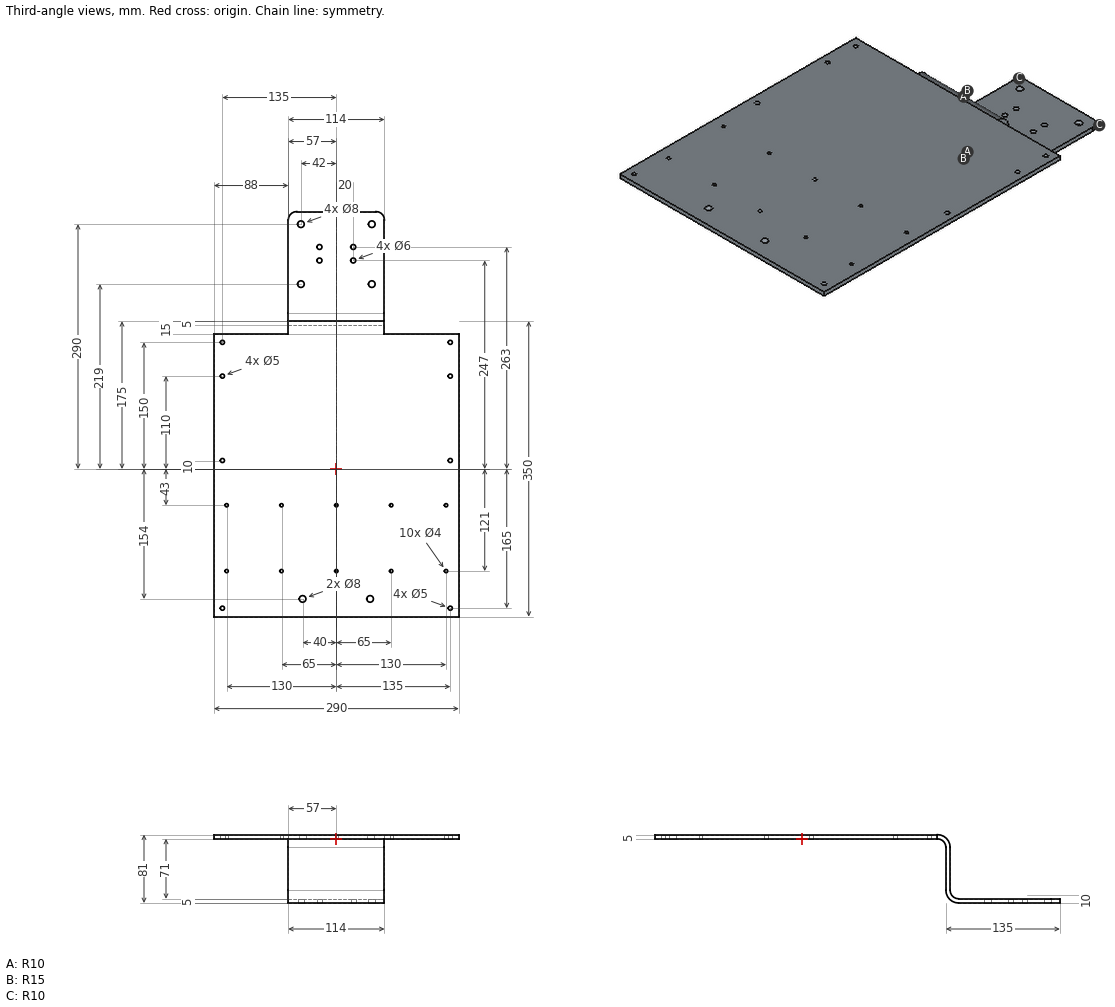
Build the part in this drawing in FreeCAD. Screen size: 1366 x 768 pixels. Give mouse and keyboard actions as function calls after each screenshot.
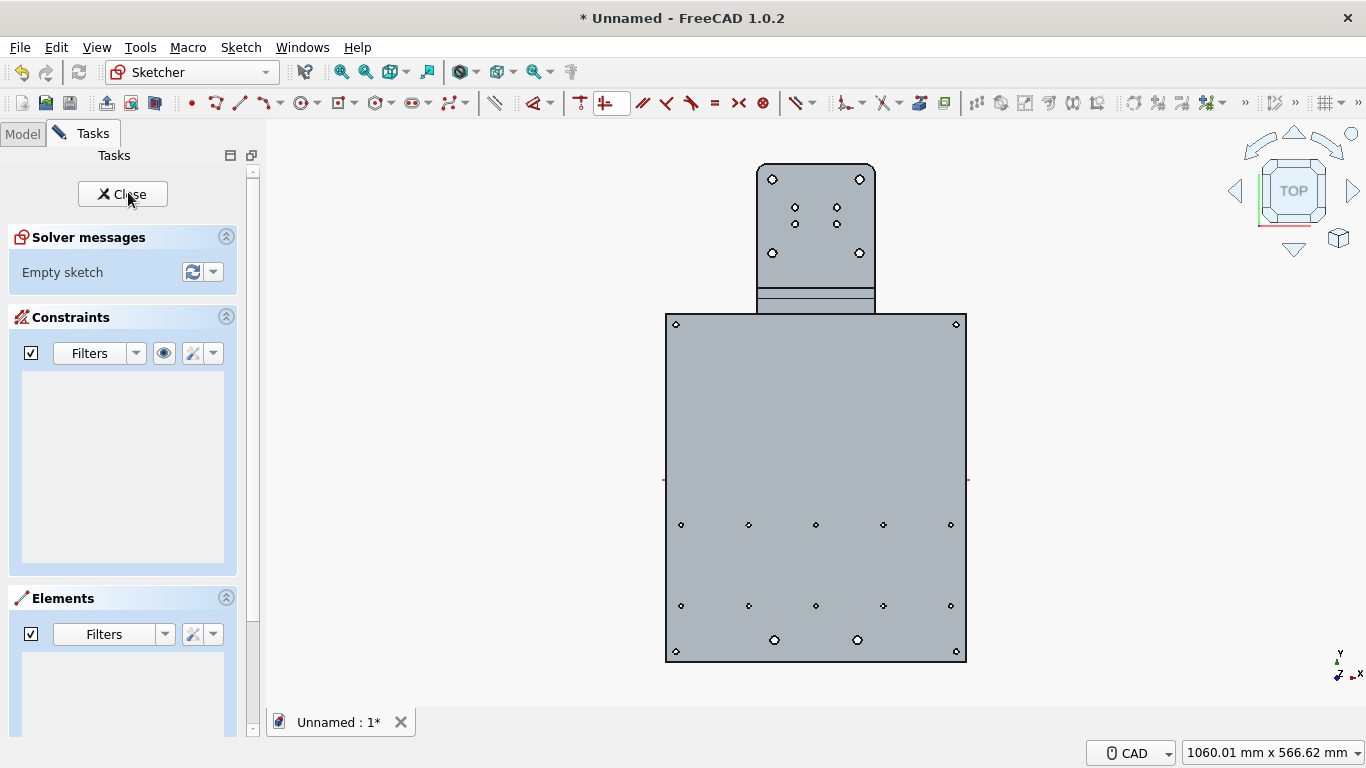
click(156, 104)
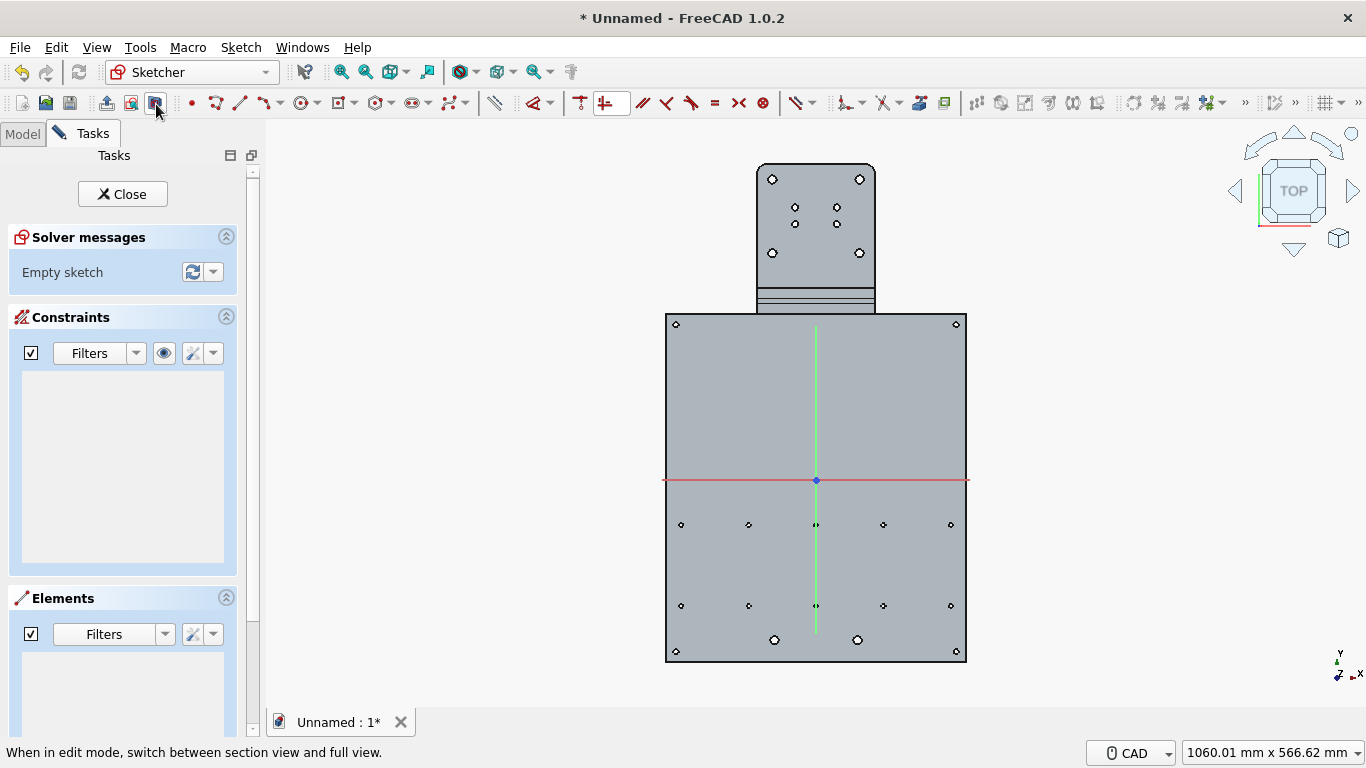
scroll(872, 429, up, 4)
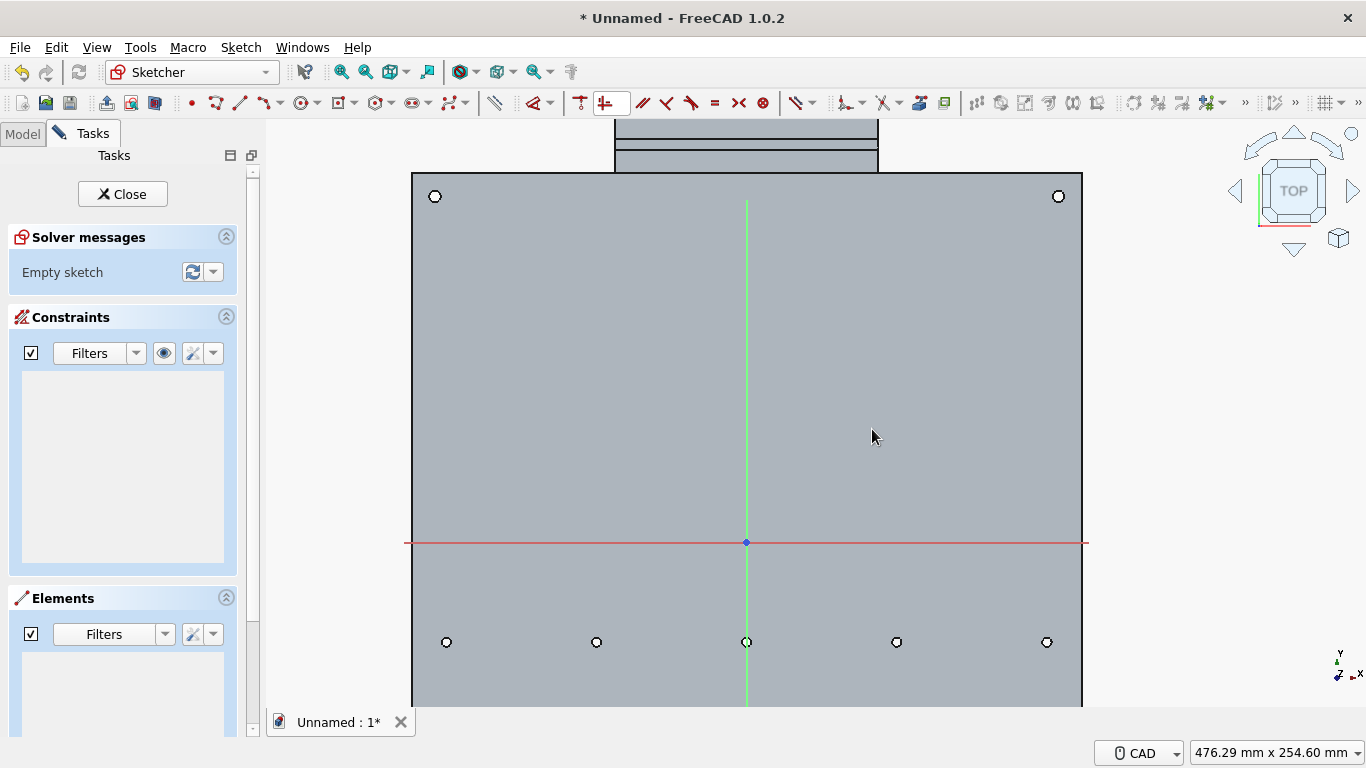
click(302, 104)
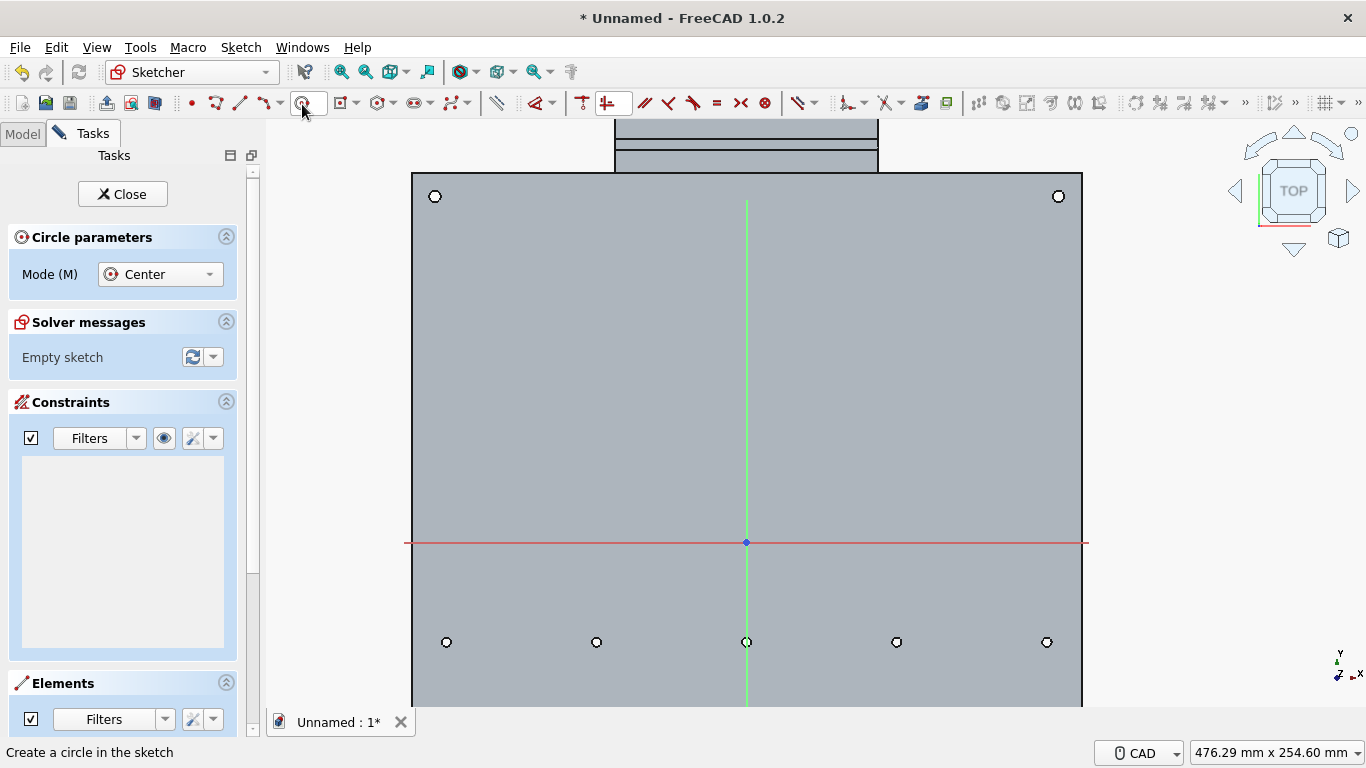
scroll(435, 289, up, 7)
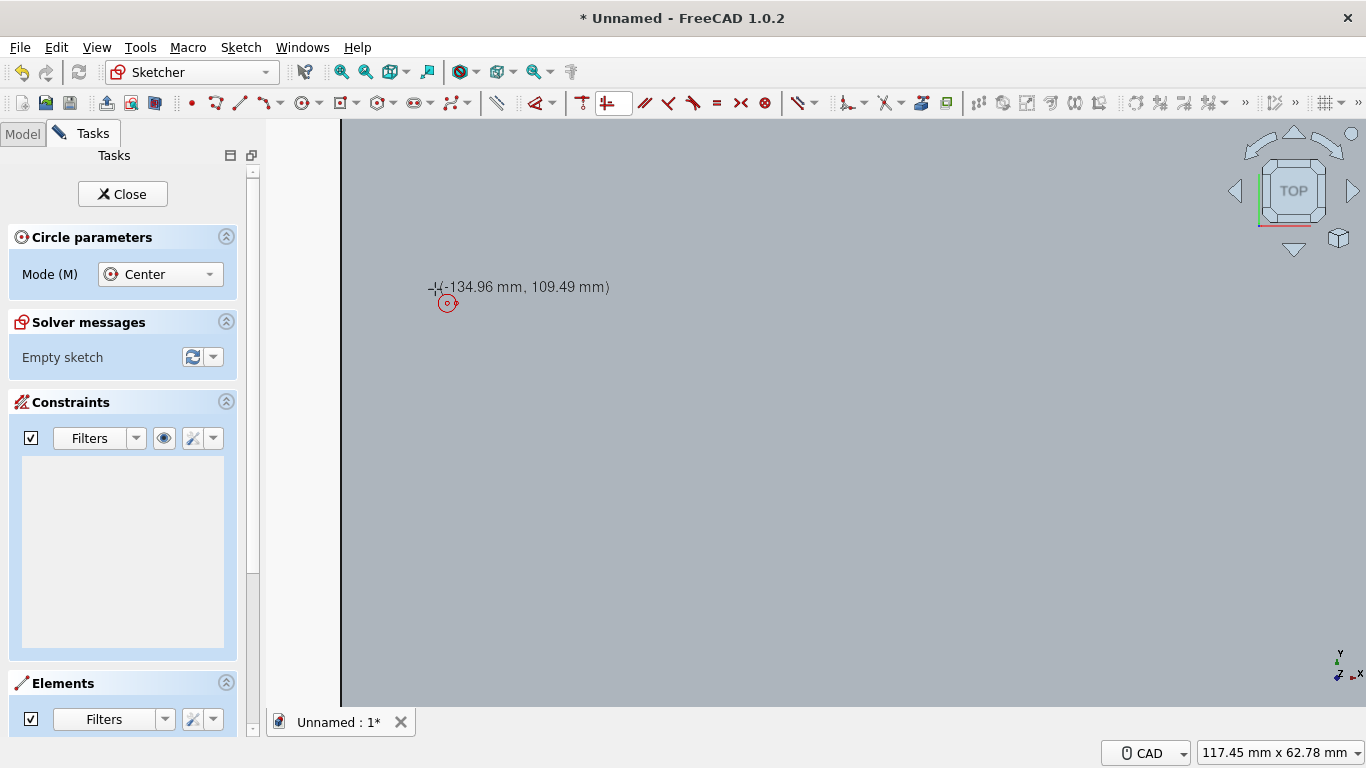
scroll(436, 289, down, 7)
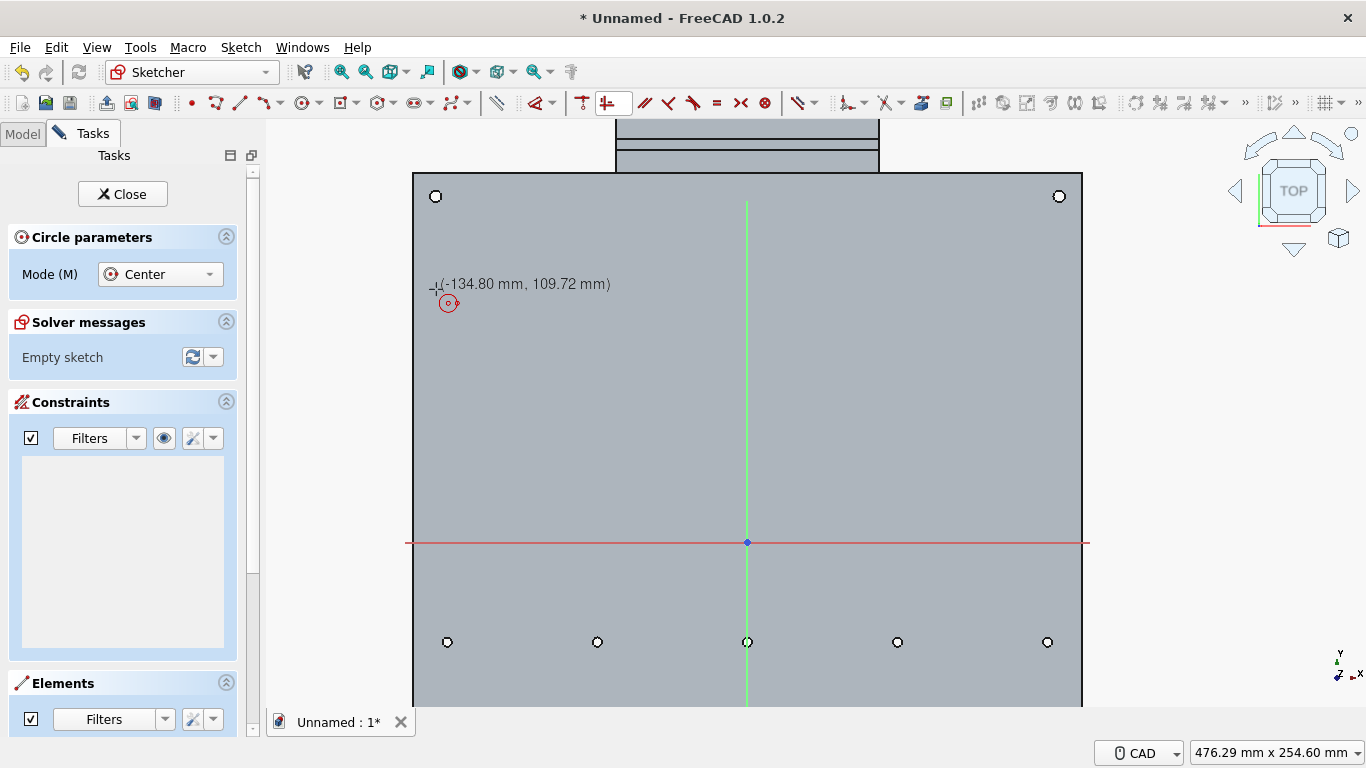
click(436, 289)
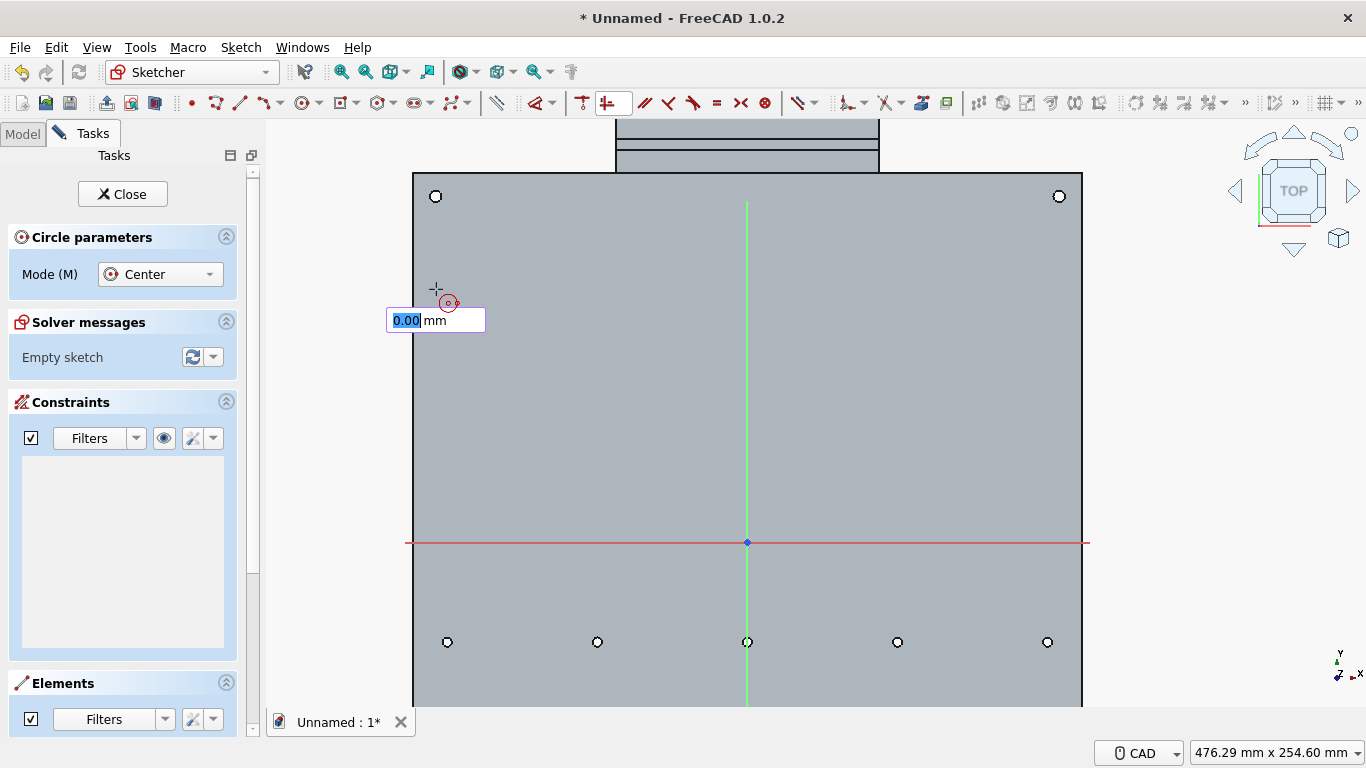
scroll(440, 285, up, 6)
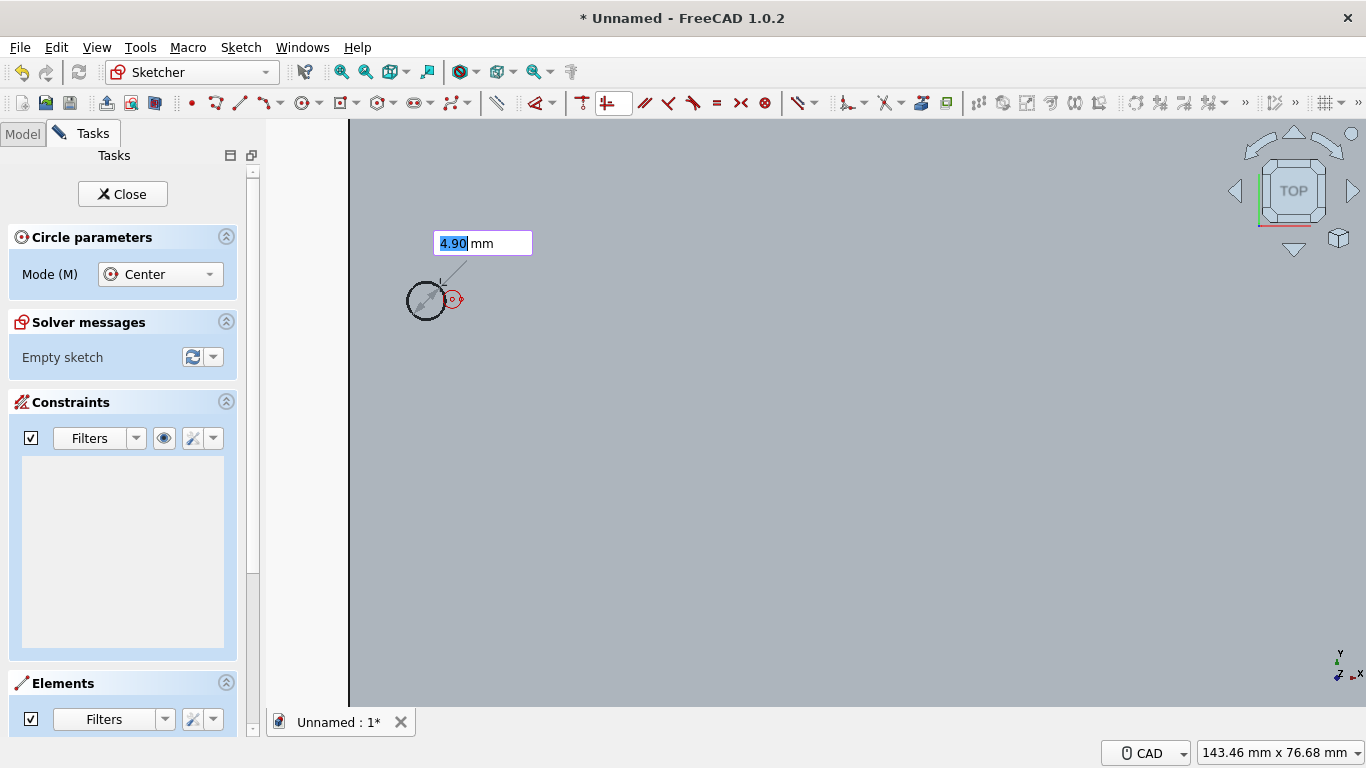
click(439, 283)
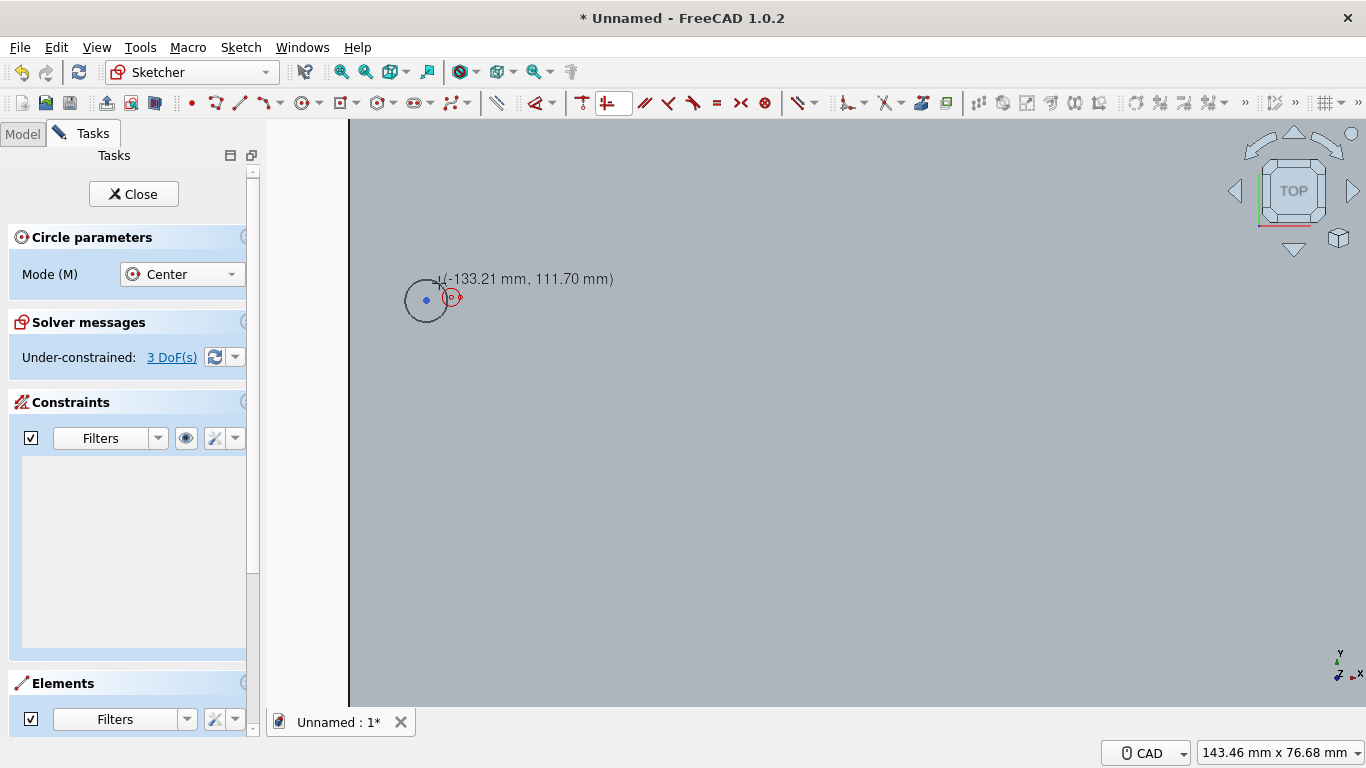
scroll(440, 285, down, 6)